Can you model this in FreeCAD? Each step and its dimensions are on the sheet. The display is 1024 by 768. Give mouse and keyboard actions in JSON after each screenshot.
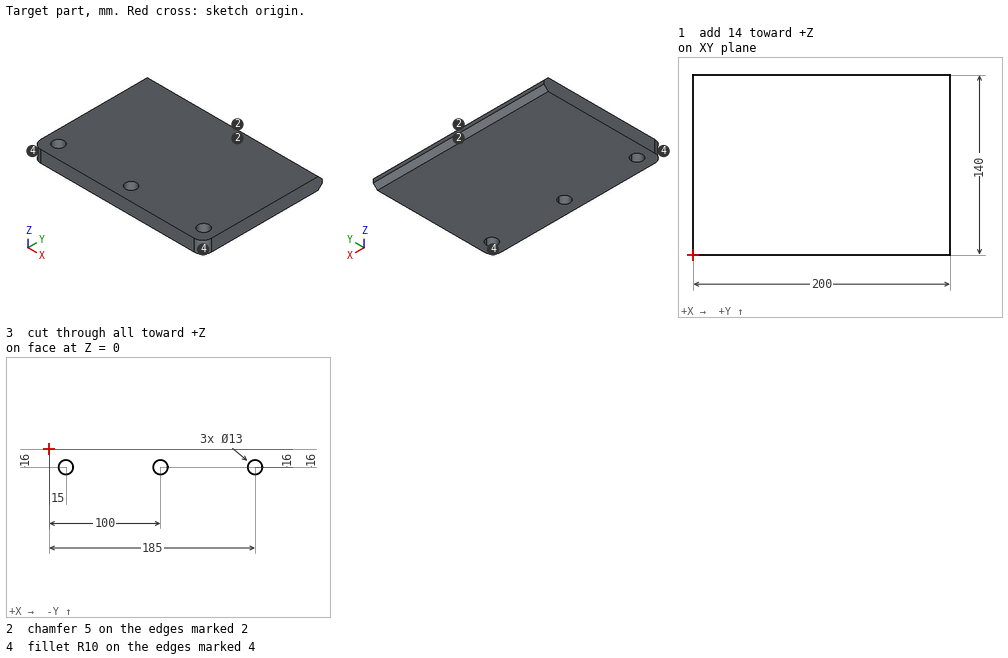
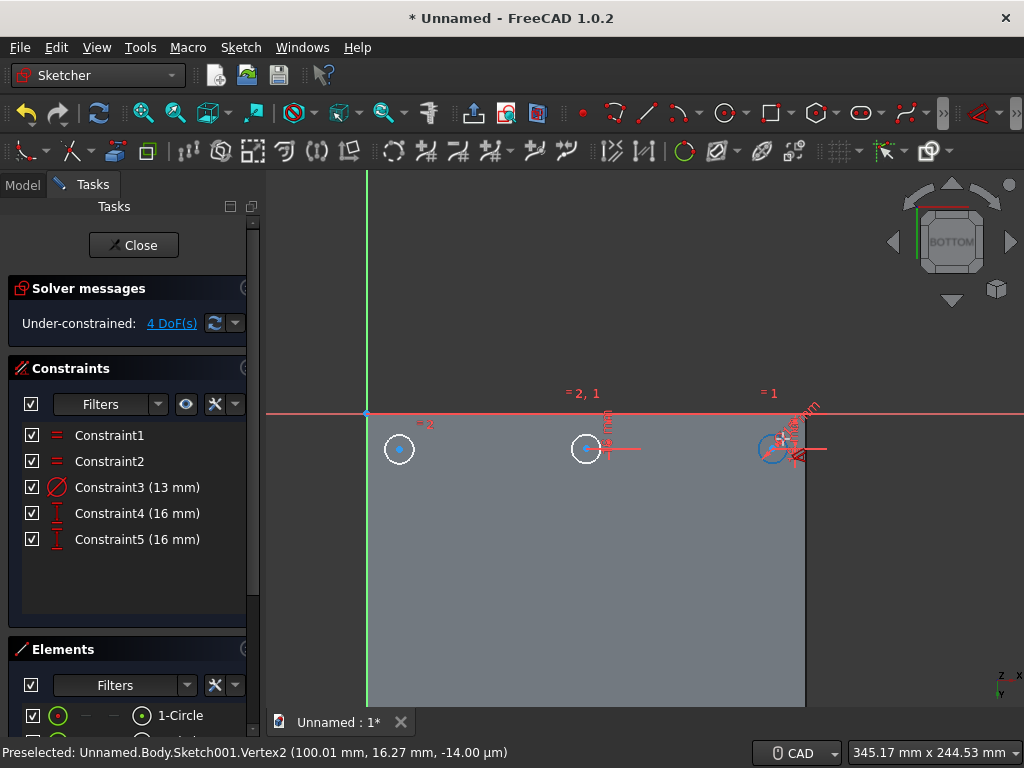
{"action": "left_click", "coordinate": [399, 449]}
{"action": "left_click", "coordinate": [383, 380]}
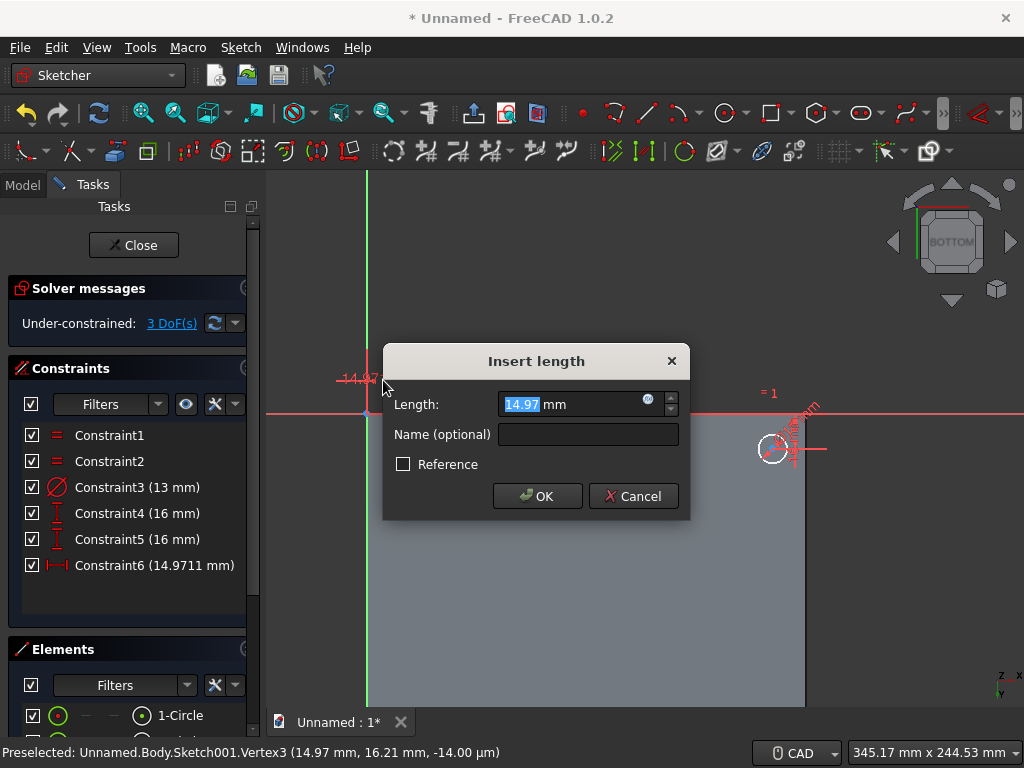
{"action": "type", "text": "15"}
{"action": "key", "text": "Return"}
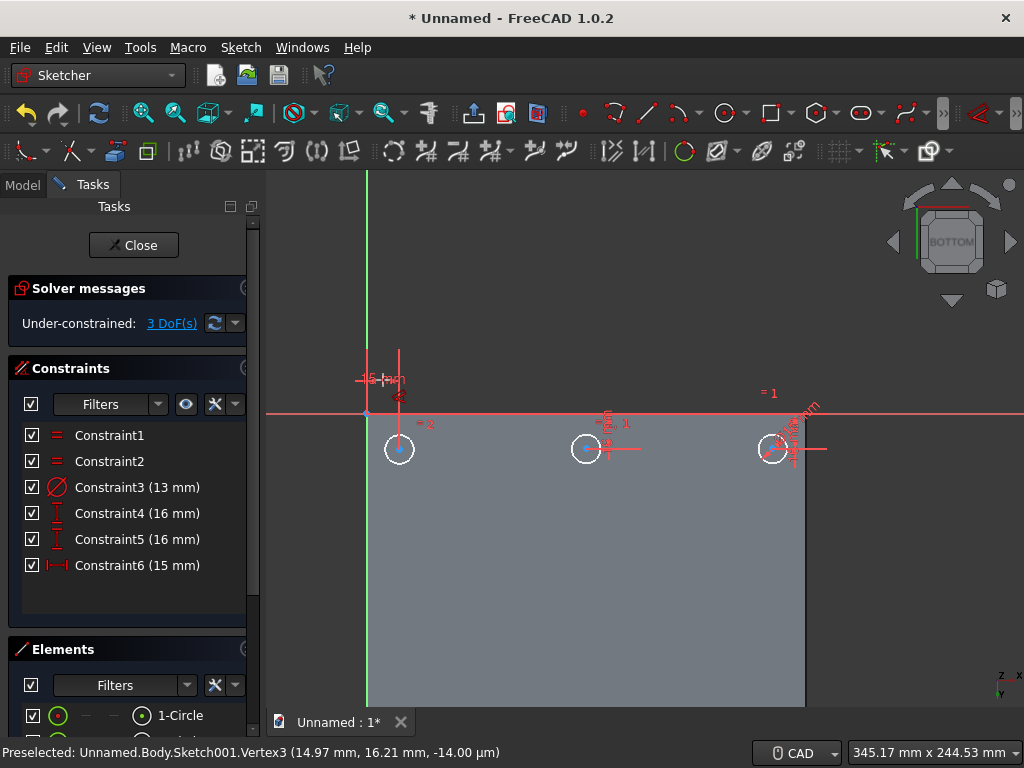
{"action": "left_click", "coordinate": [399, 449]}
{"action": "left_click", "coordinate": [333, 432]}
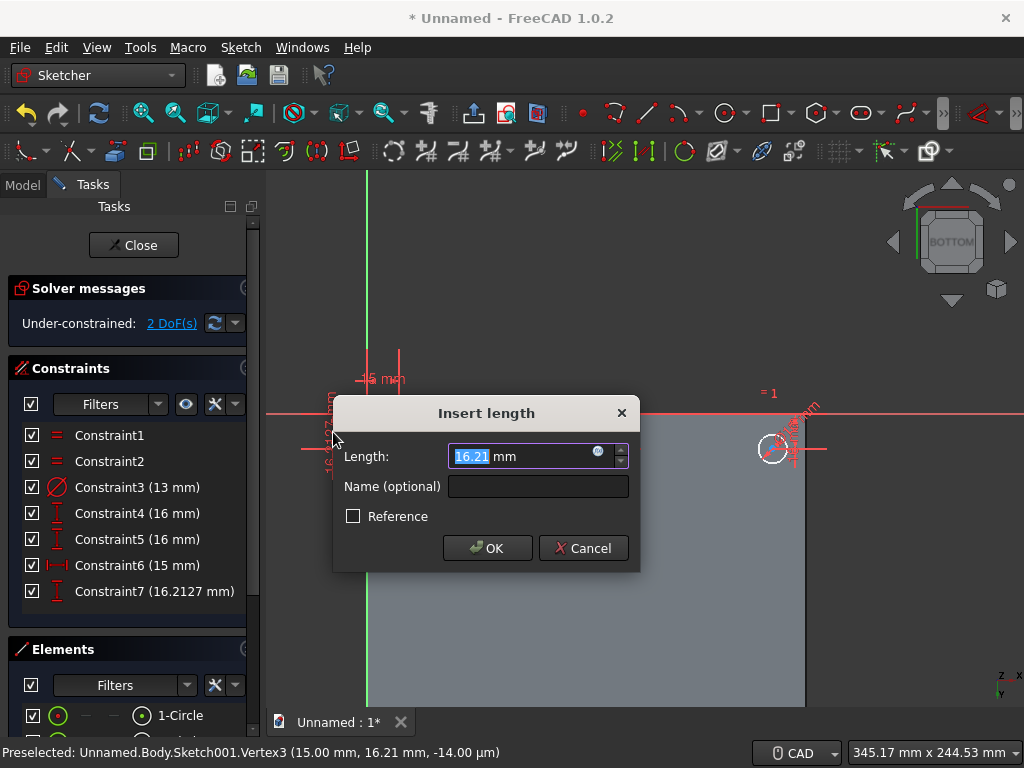
{"action": "type", "text": "16"}
{"action": "key", "text": "Return"}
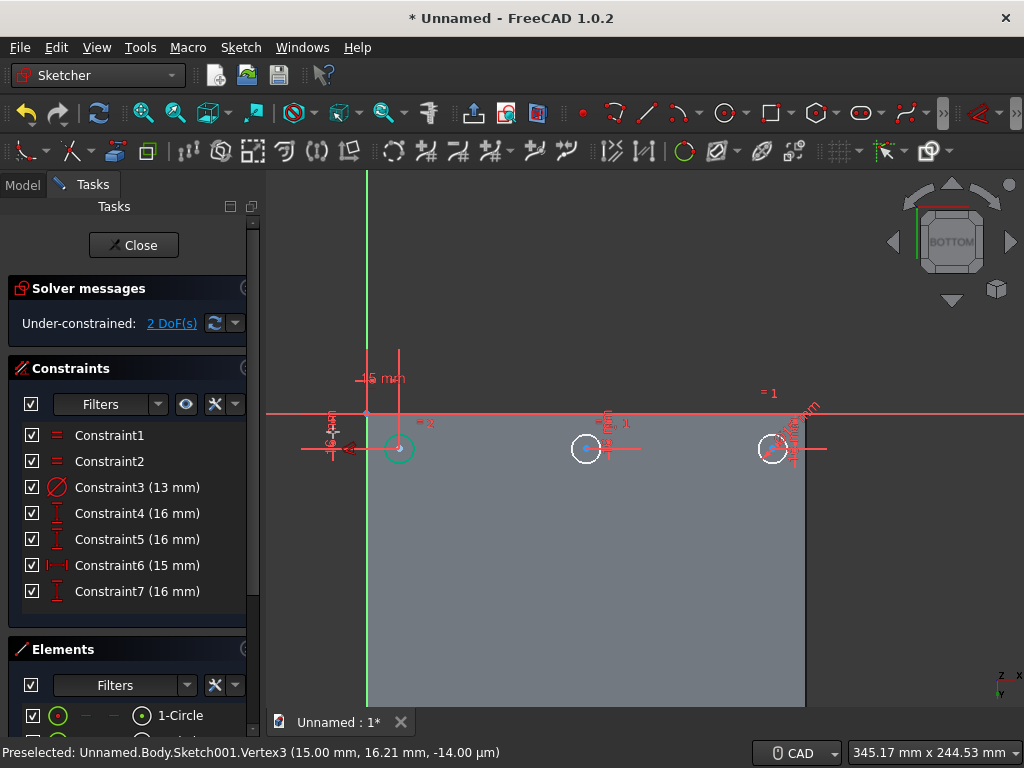
{"action": "left_click", "coordinate": [773, 449]}
{"action": "left_click", "coordinate": [570, 380]}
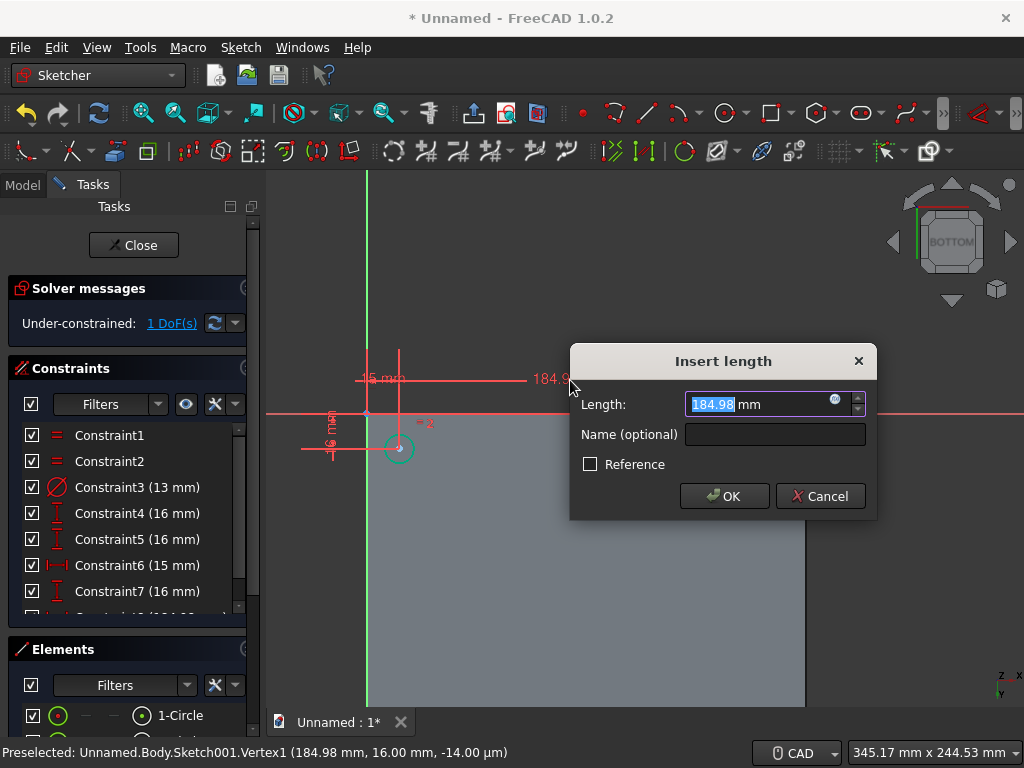
{"action": "type", "text": "185"}
{"action": "key", "text": "Return"}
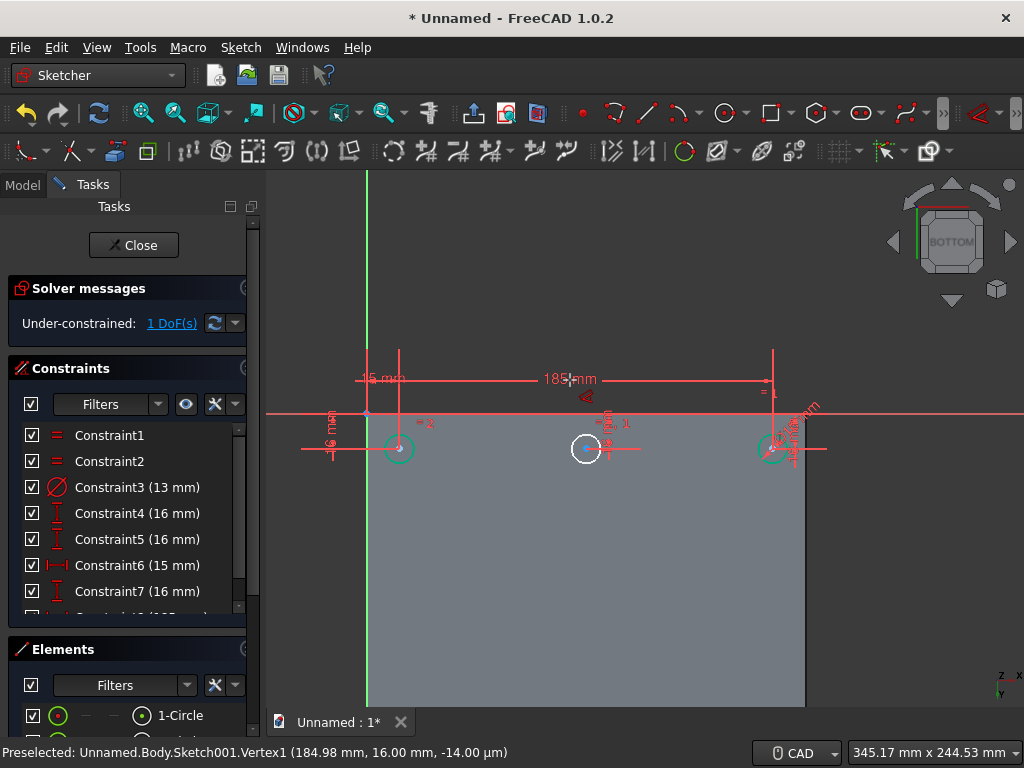
{"action": "left_click", "coordinate": [586, 449]}
{"action": "left_click", "coordinate": [476, 380]}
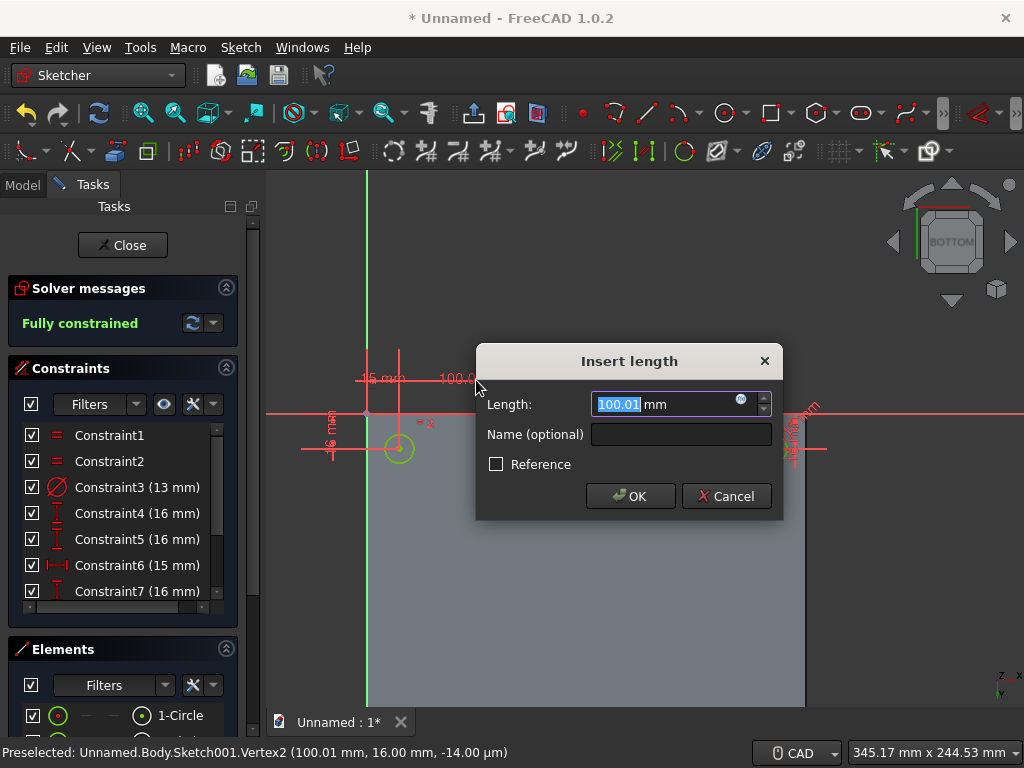
{"action": "type", "text": "100"}
{"action": "key", "text": "Return"}
{"action": "key", "text": "Escape"}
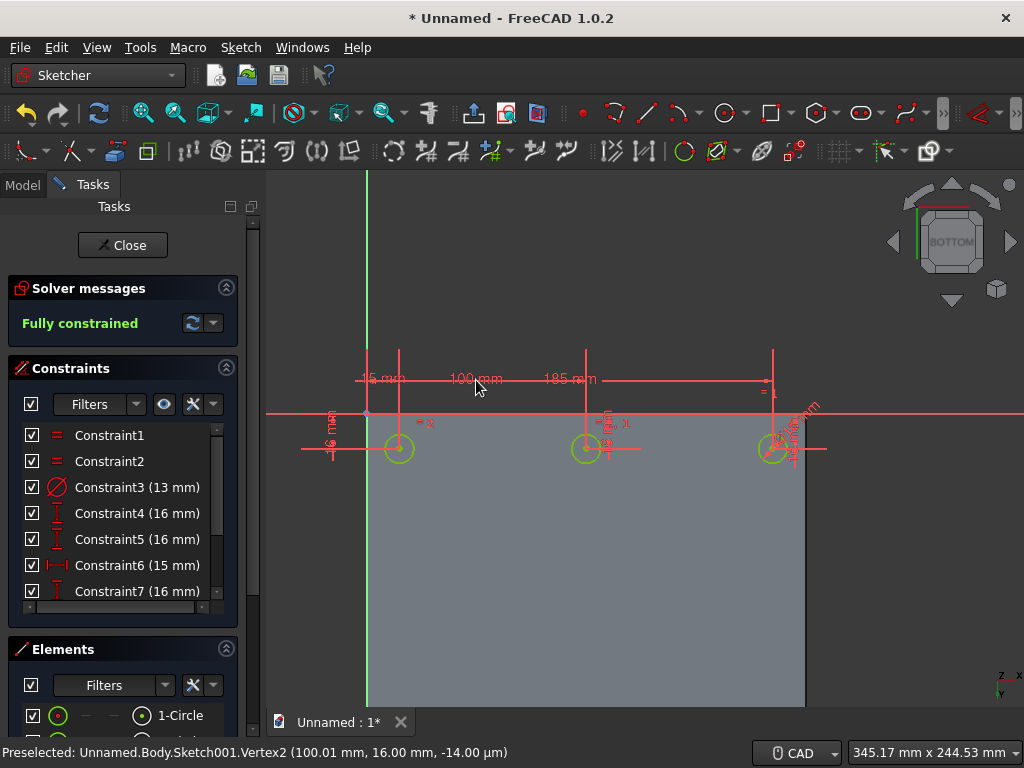
{"action": "left_click", "coordinate": [123, 245]}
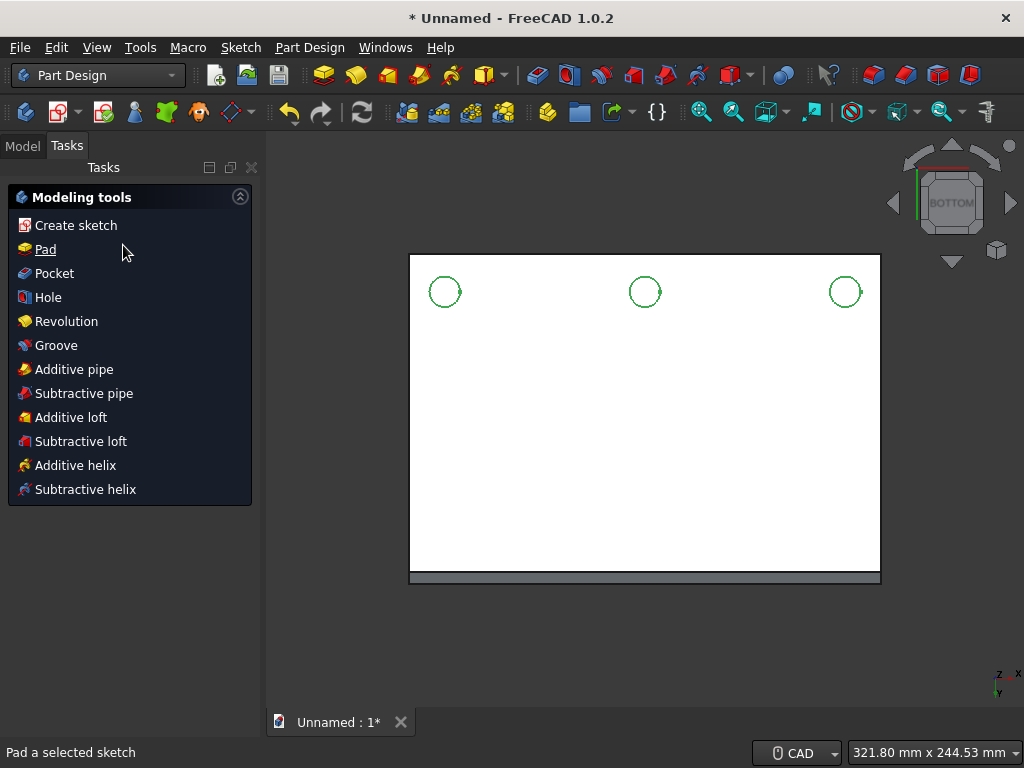
{"action": "left_click", "coordinate": [538, 76]}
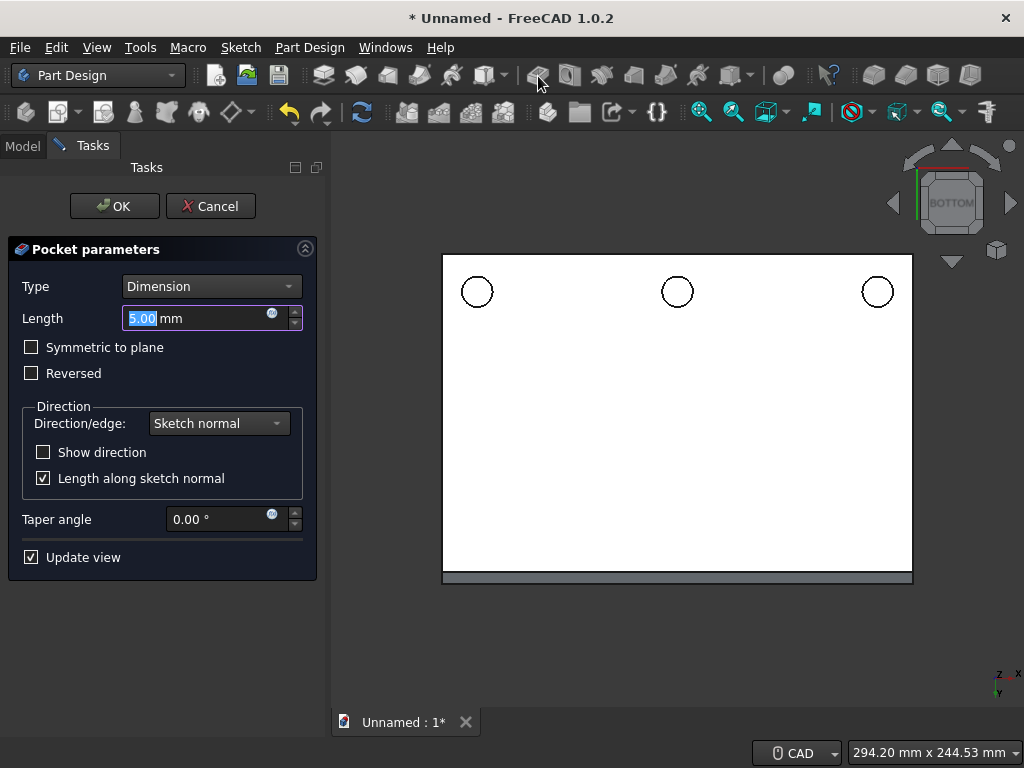
{"action": "left_click", "coordinate": [212, 286]}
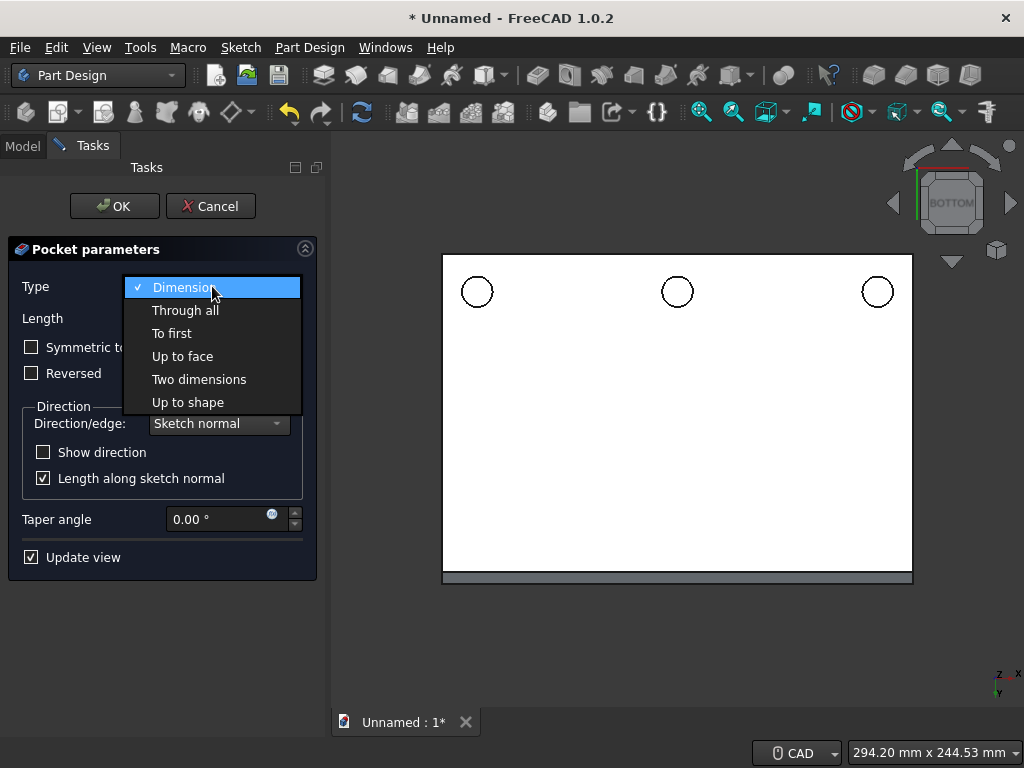
{"action": "left_click", "coordinate": [212, 310]}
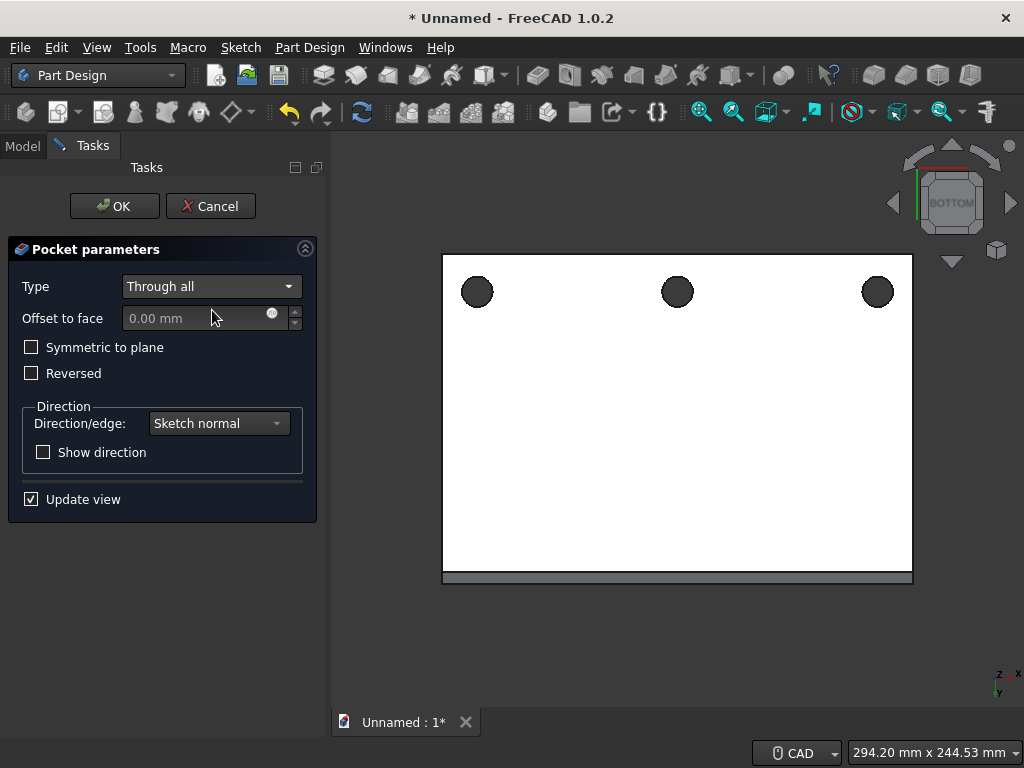
{"action": "left_click", "coordinate": [115, 206]}